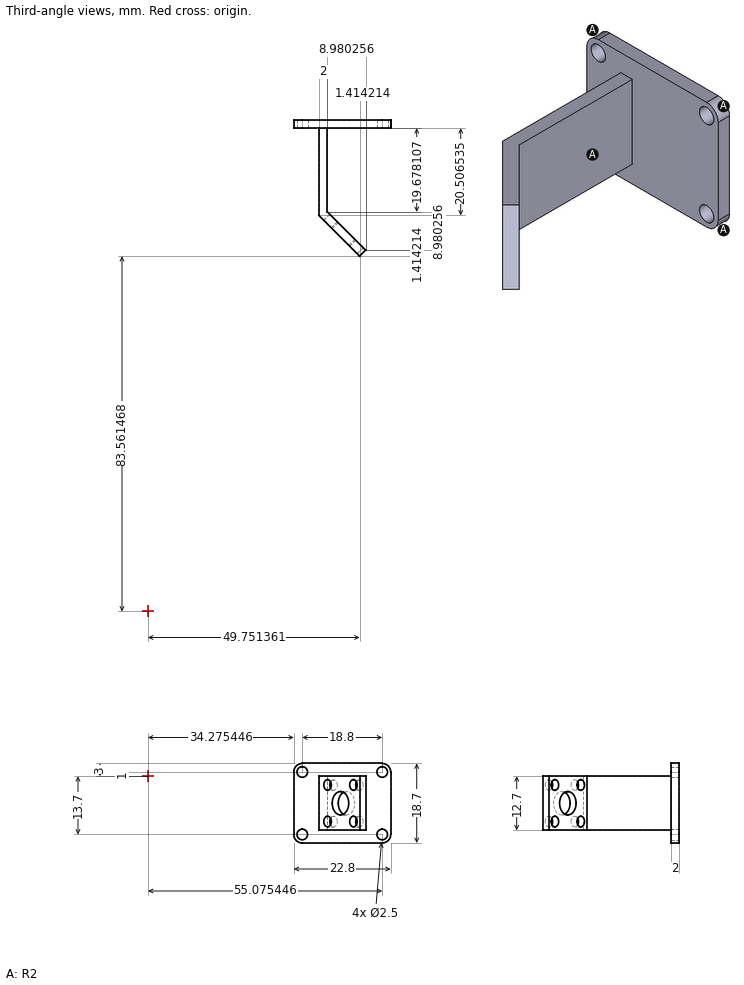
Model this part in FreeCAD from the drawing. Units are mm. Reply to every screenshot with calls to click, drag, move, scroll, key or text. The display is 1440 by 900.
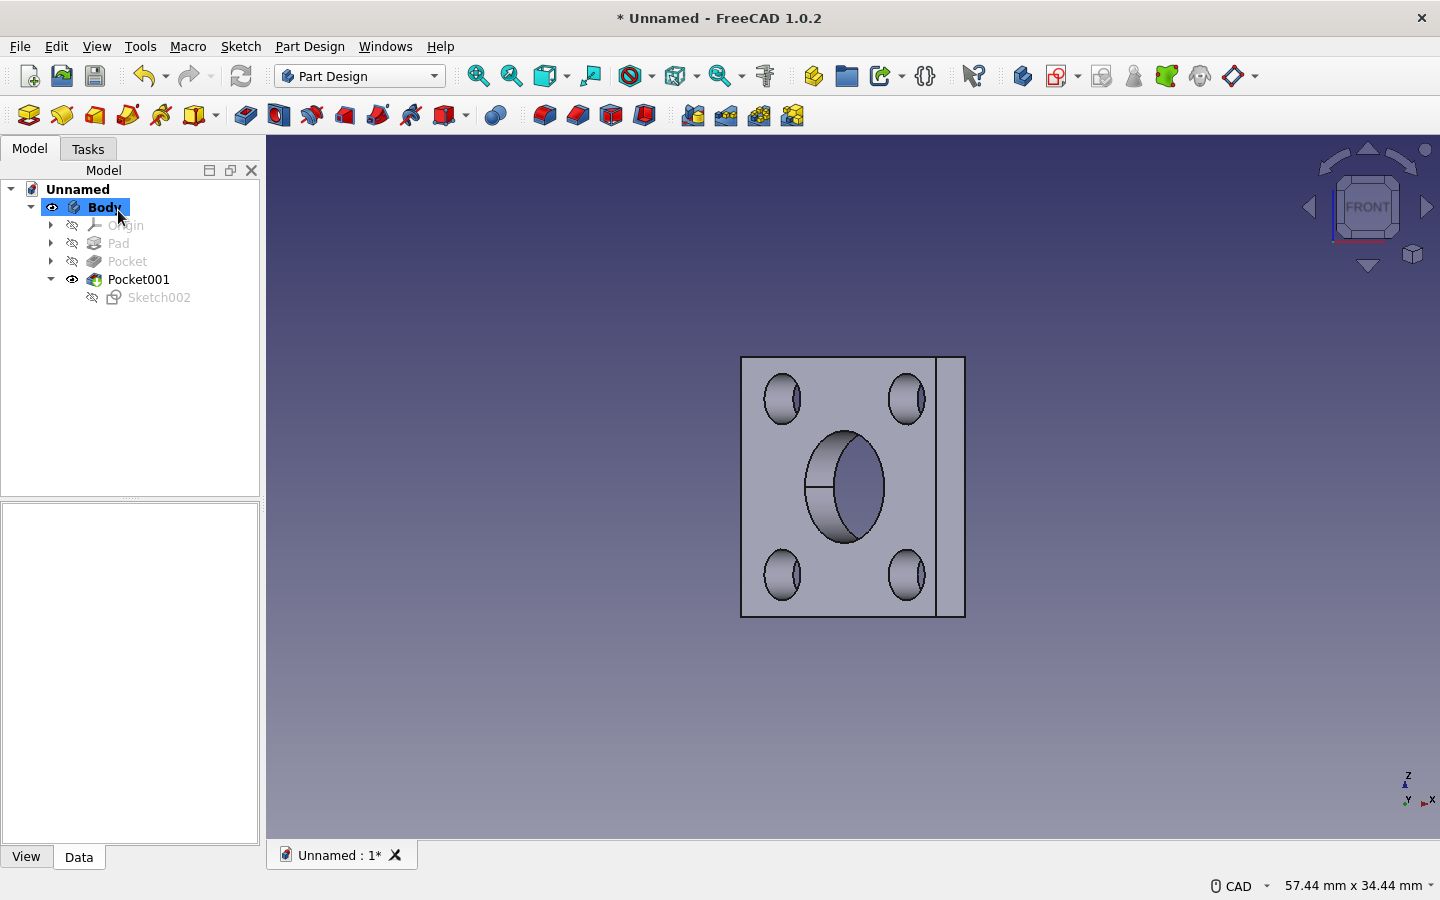
click(479, 76)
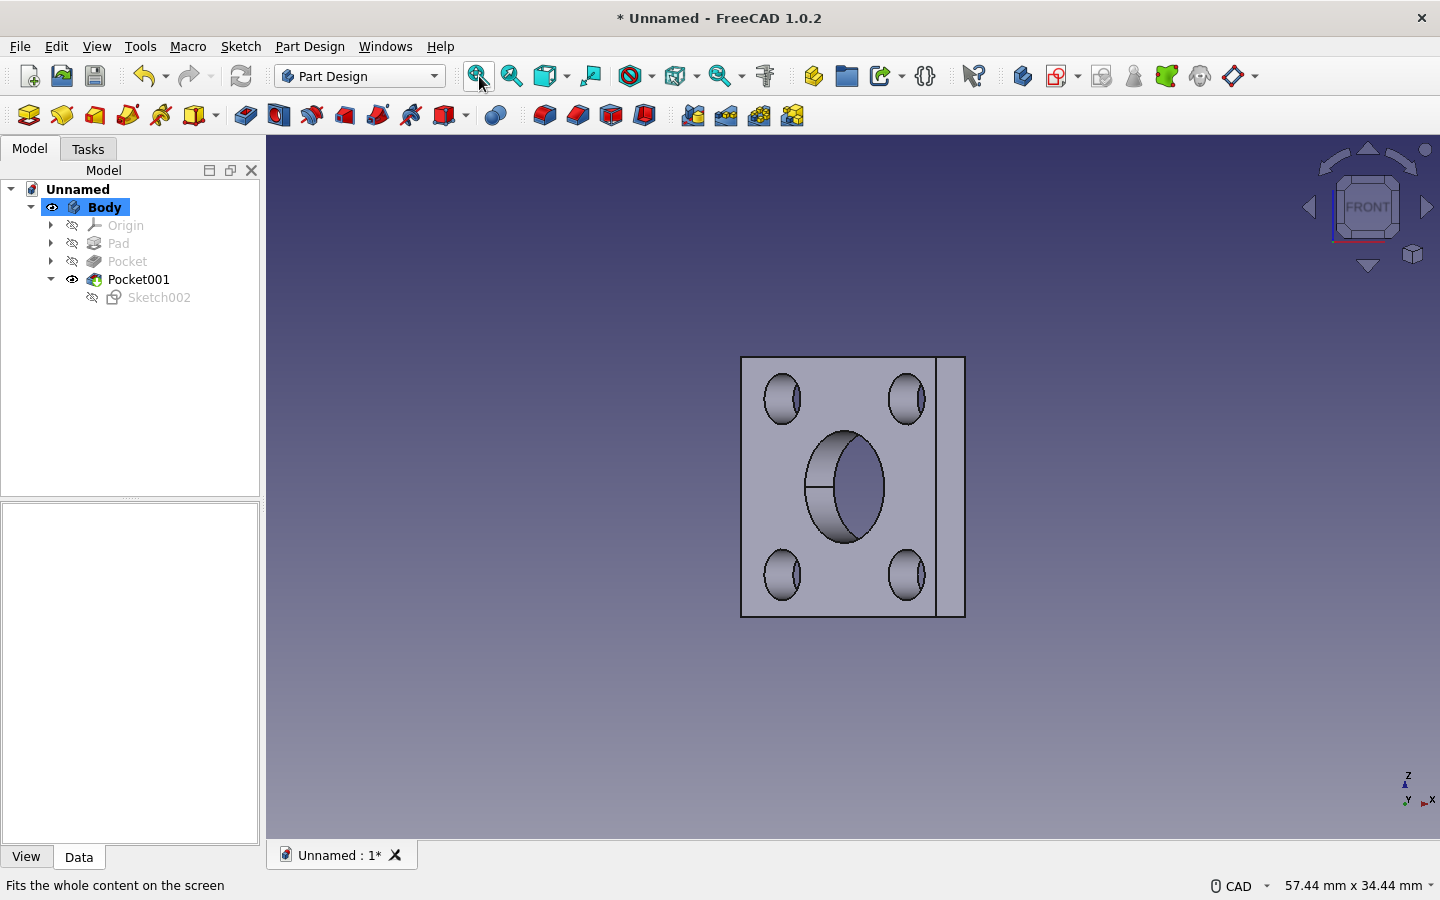
click(1023, 76)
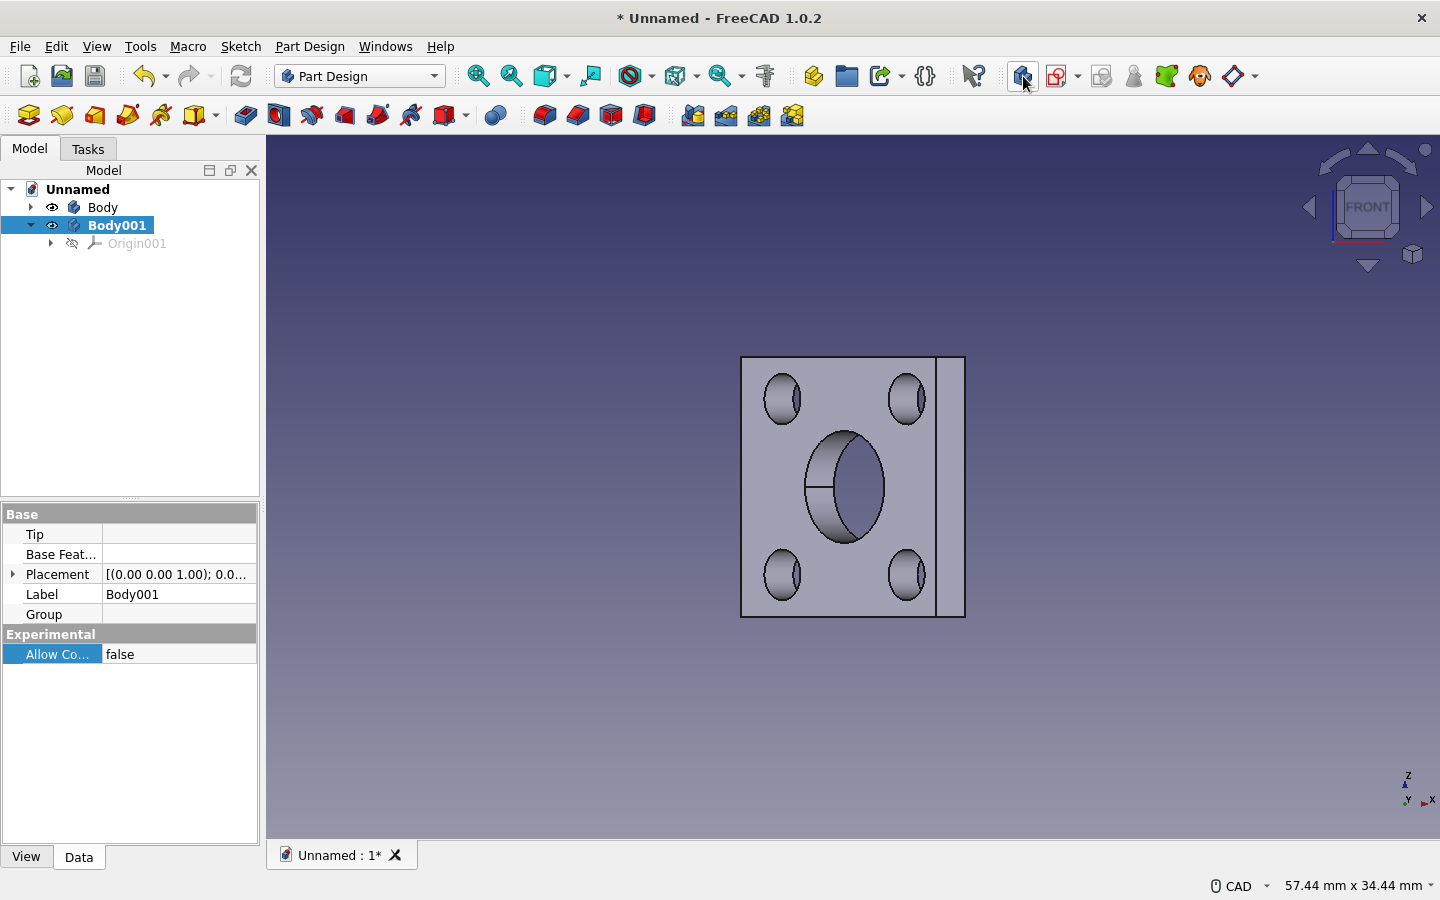
click(51, 243)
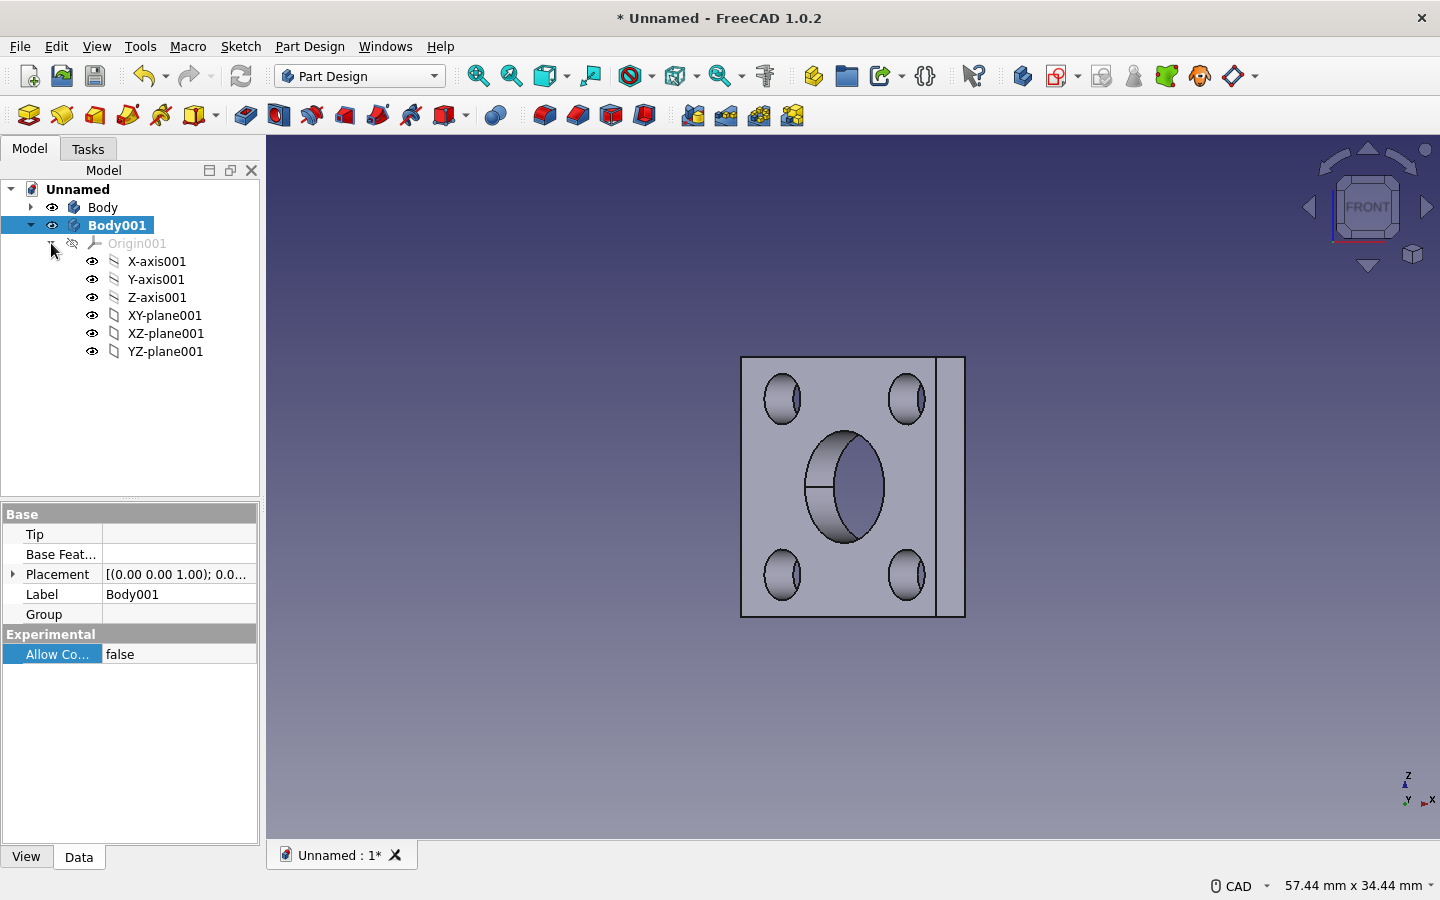
click(137, 333)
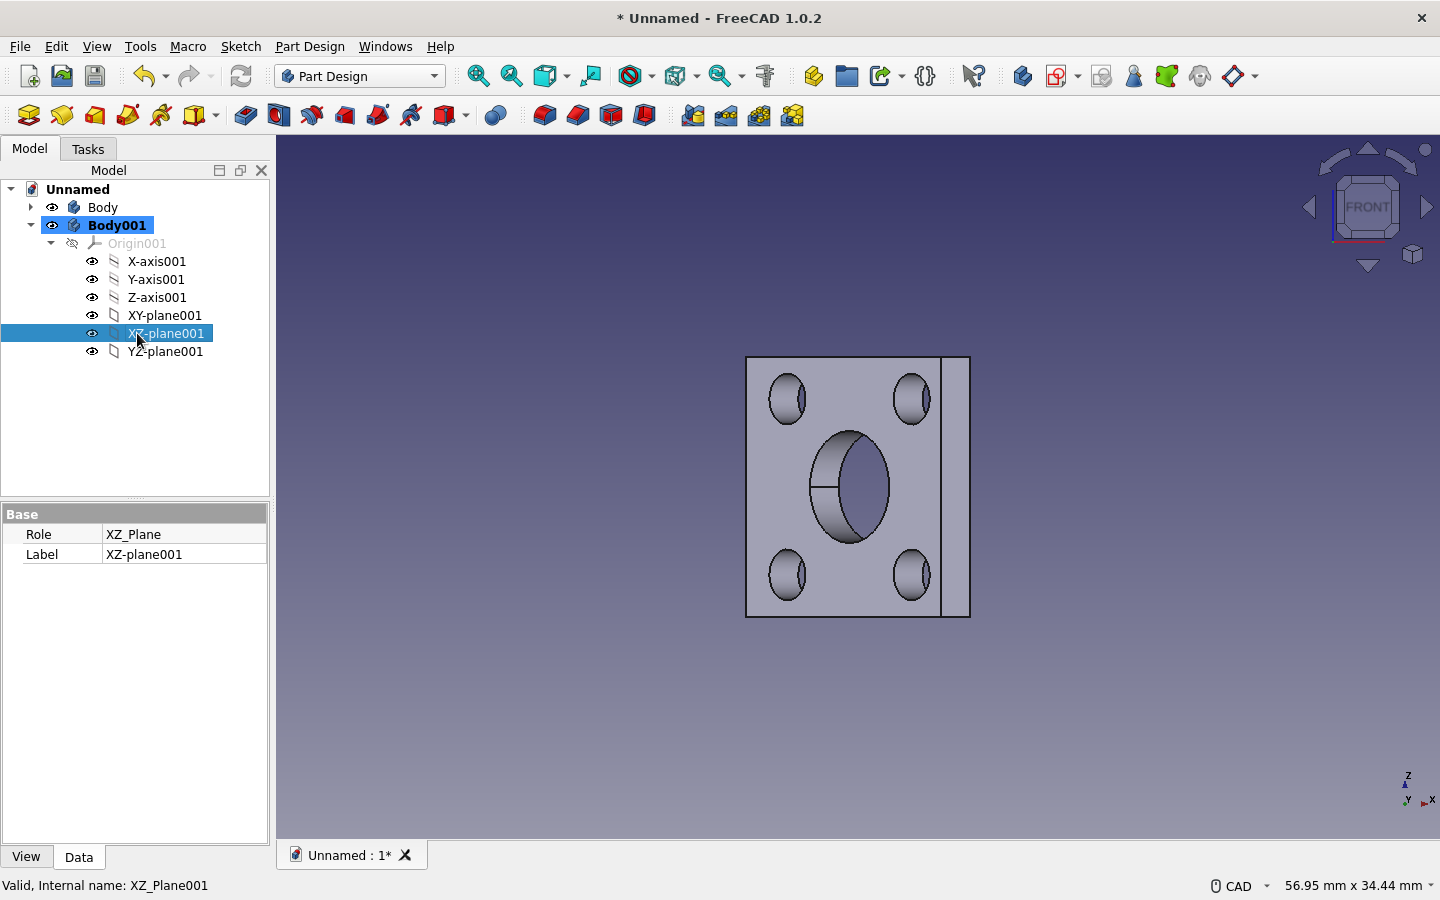
click(1232, 76)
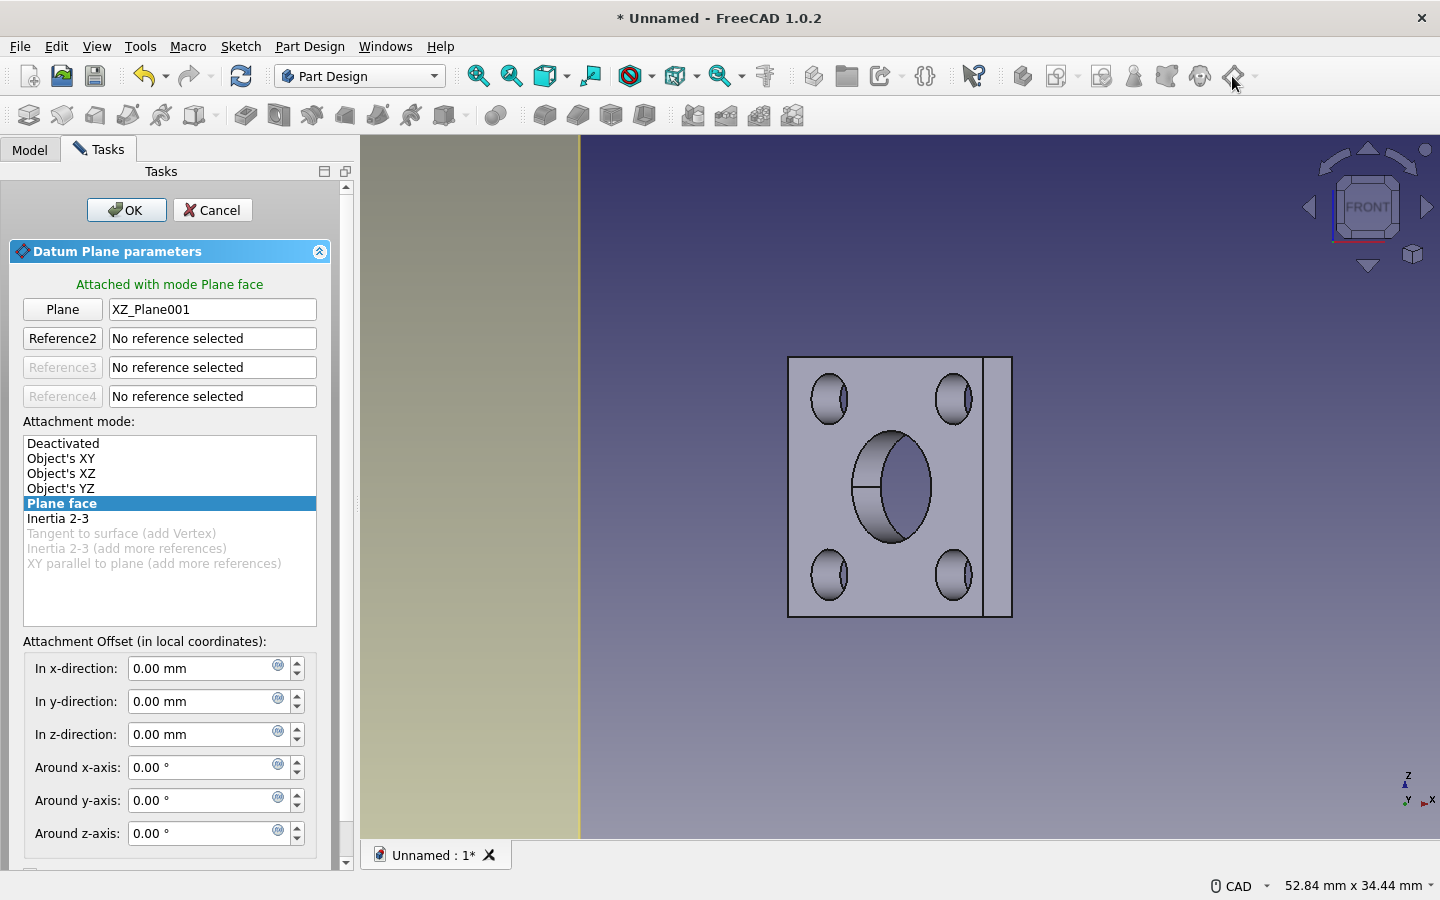
triple_click(210, 734)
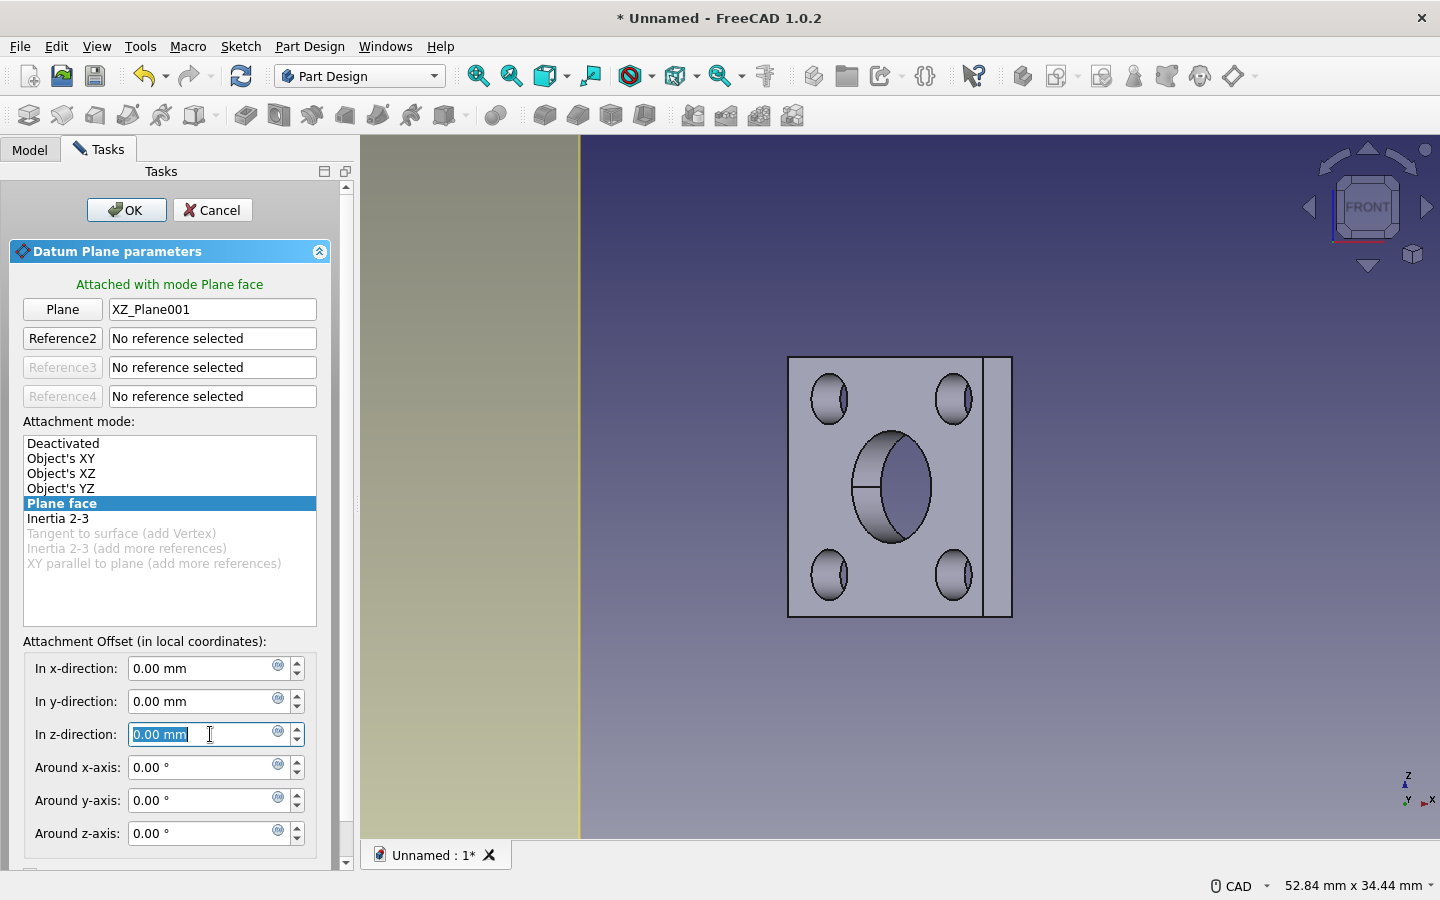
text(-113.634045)
key(Tab)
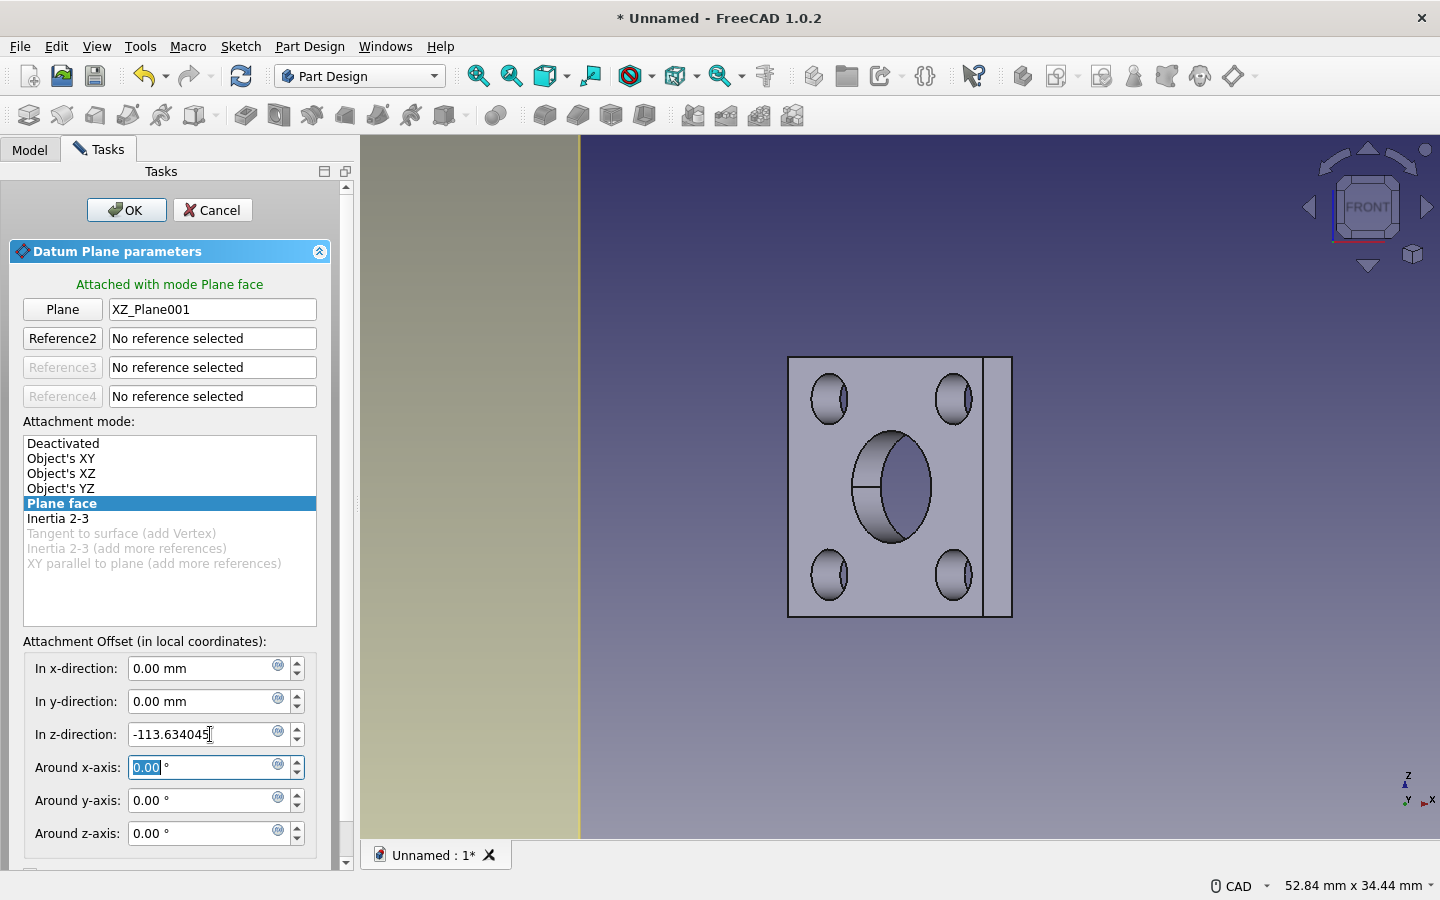
click(127, 210)